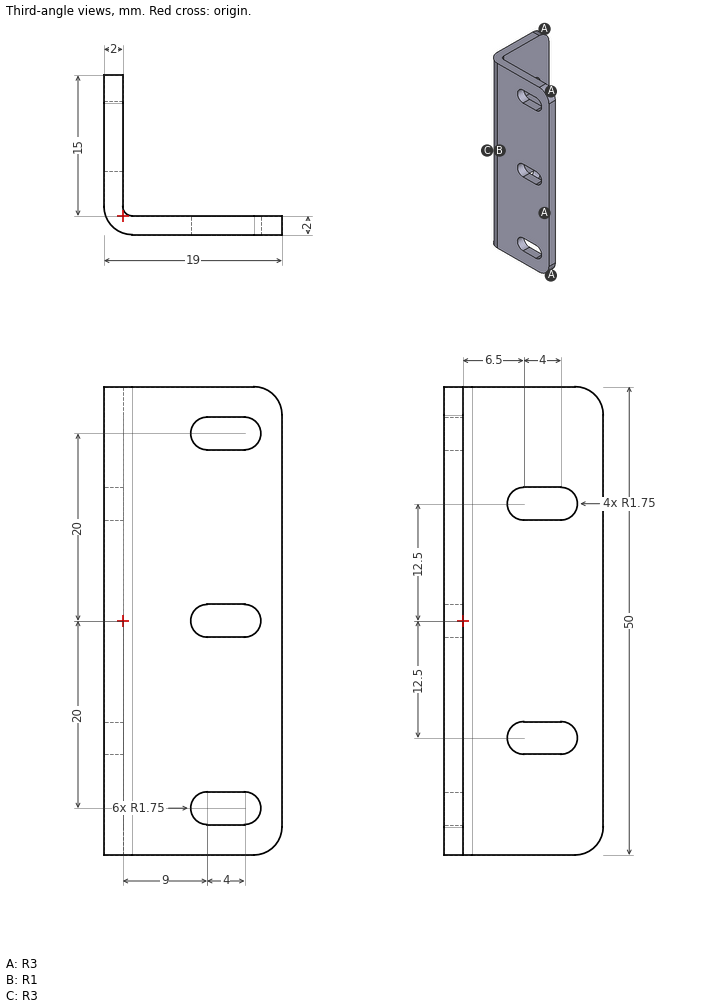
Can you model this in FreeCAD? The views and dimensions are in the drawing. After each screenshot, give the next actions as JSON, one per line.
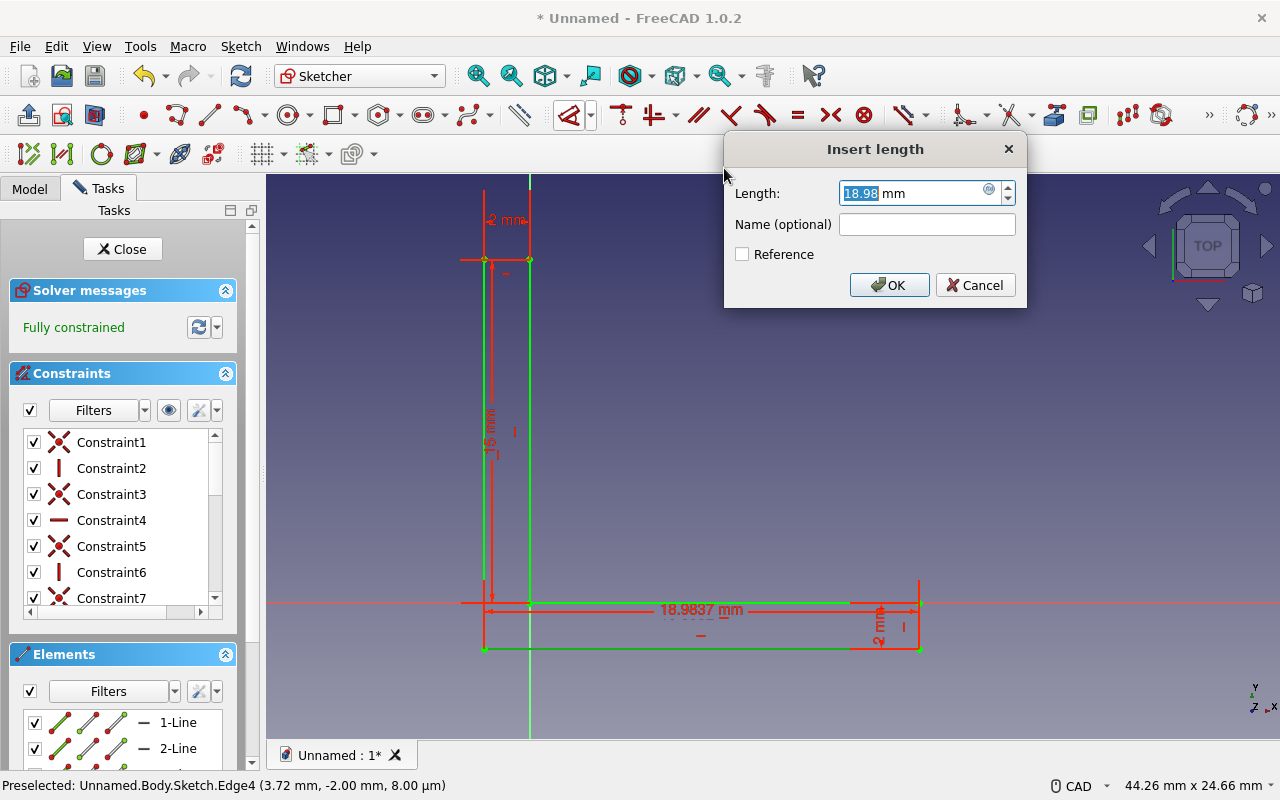
{"action": "type", "text": "19"}
{"action": "key", "text": "Return"}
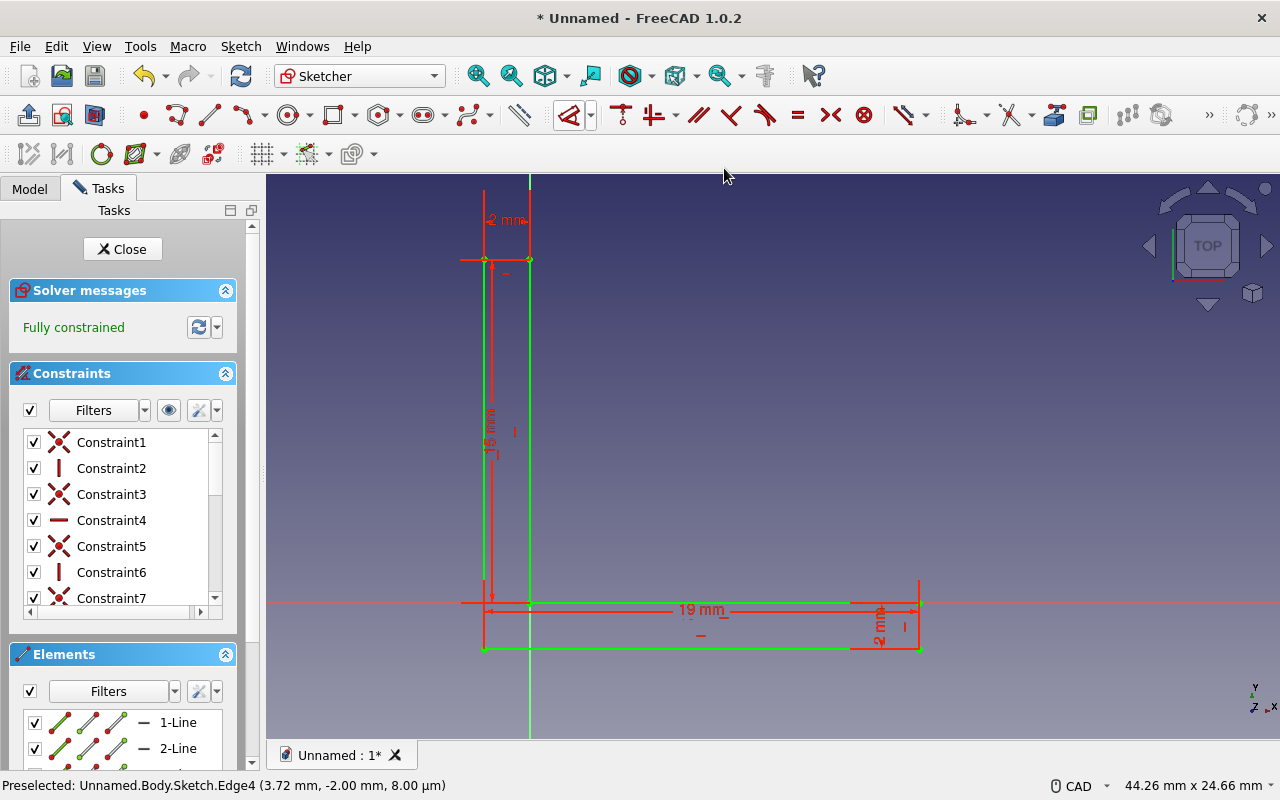
{"action": "left_click", "coordinate": [123, 249]}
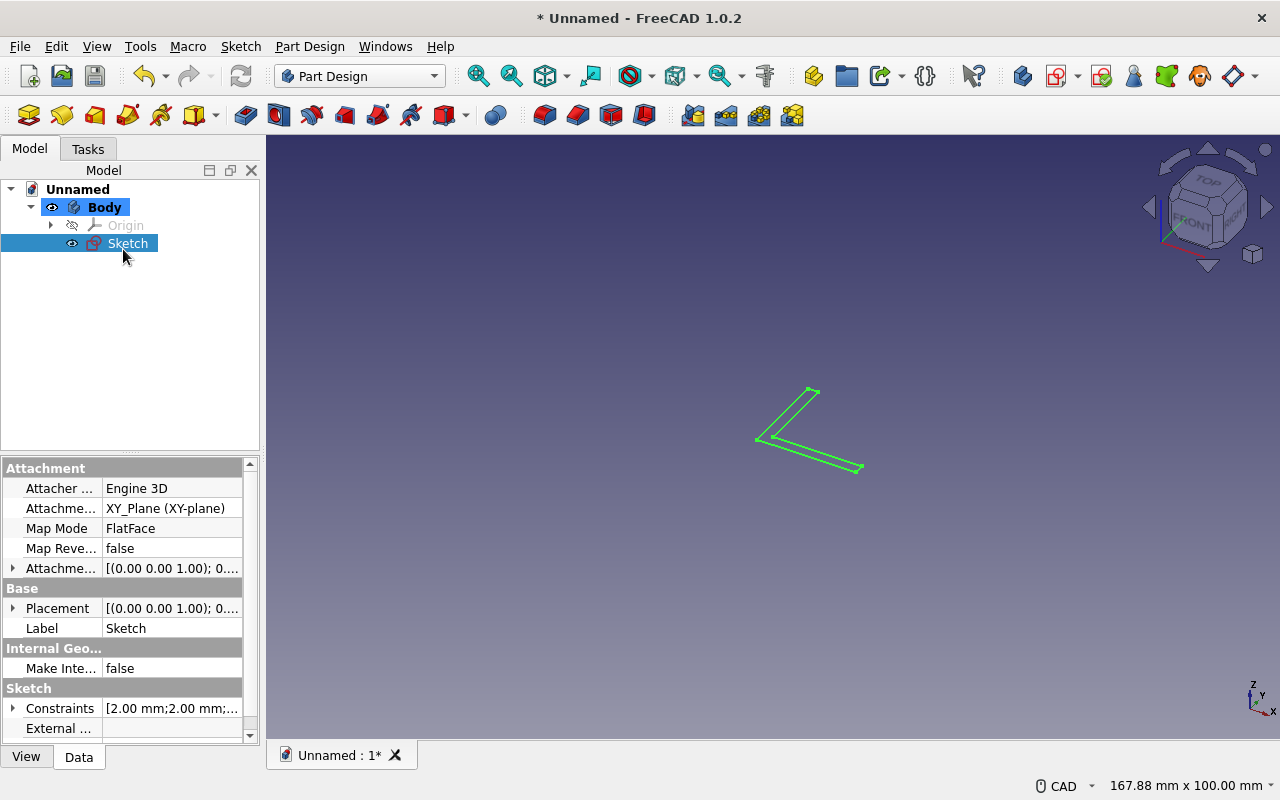
{"action": "left_click", "coordinate": [29, 116]}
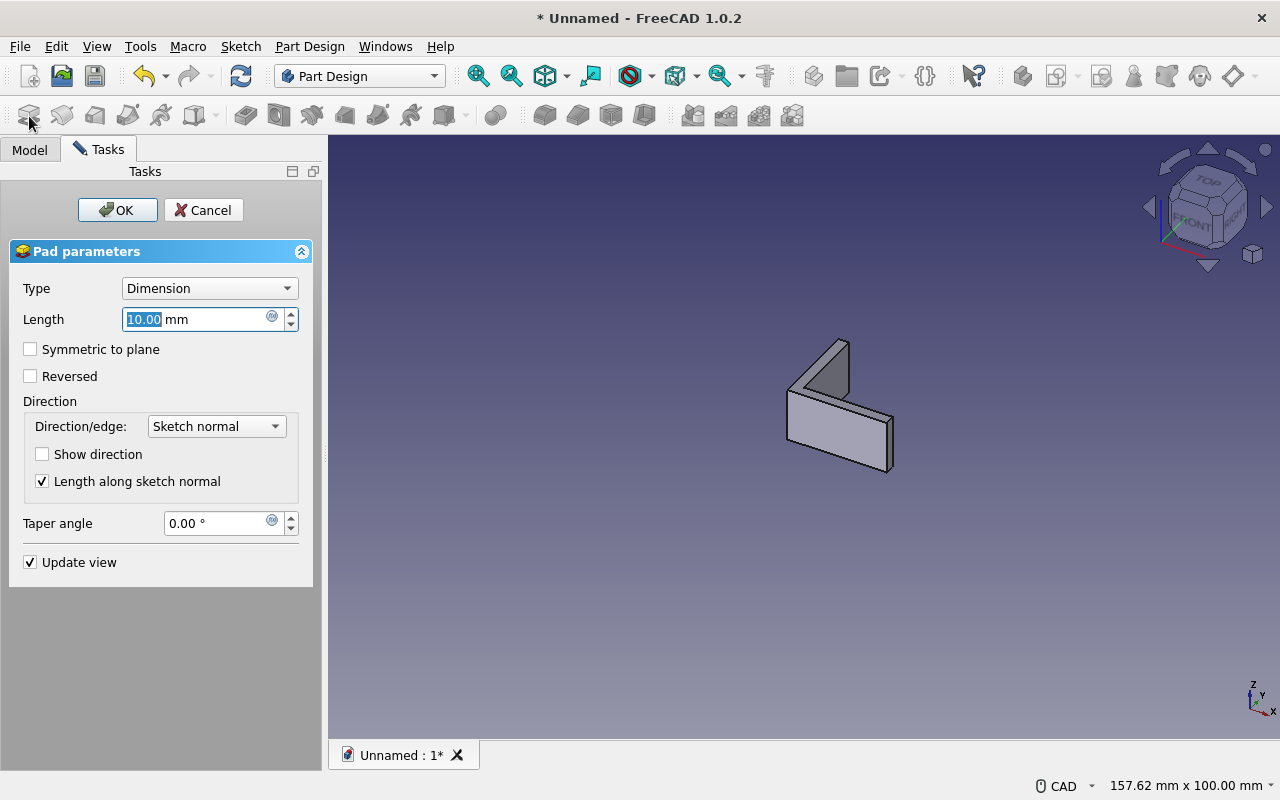
{"action": "type", "text": "50"}
{"action": "key", "text": "Tab"}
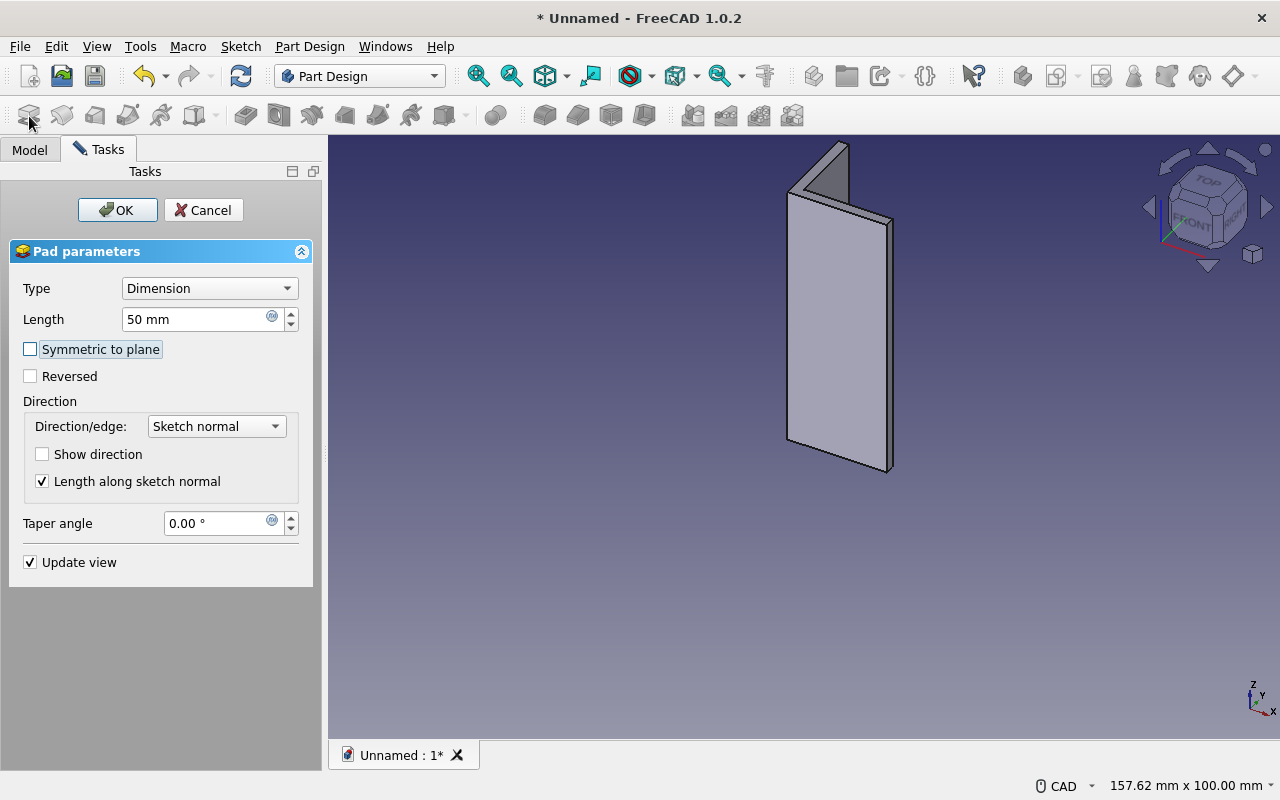
{"action": "left_click", "coordinate": [31, 349]}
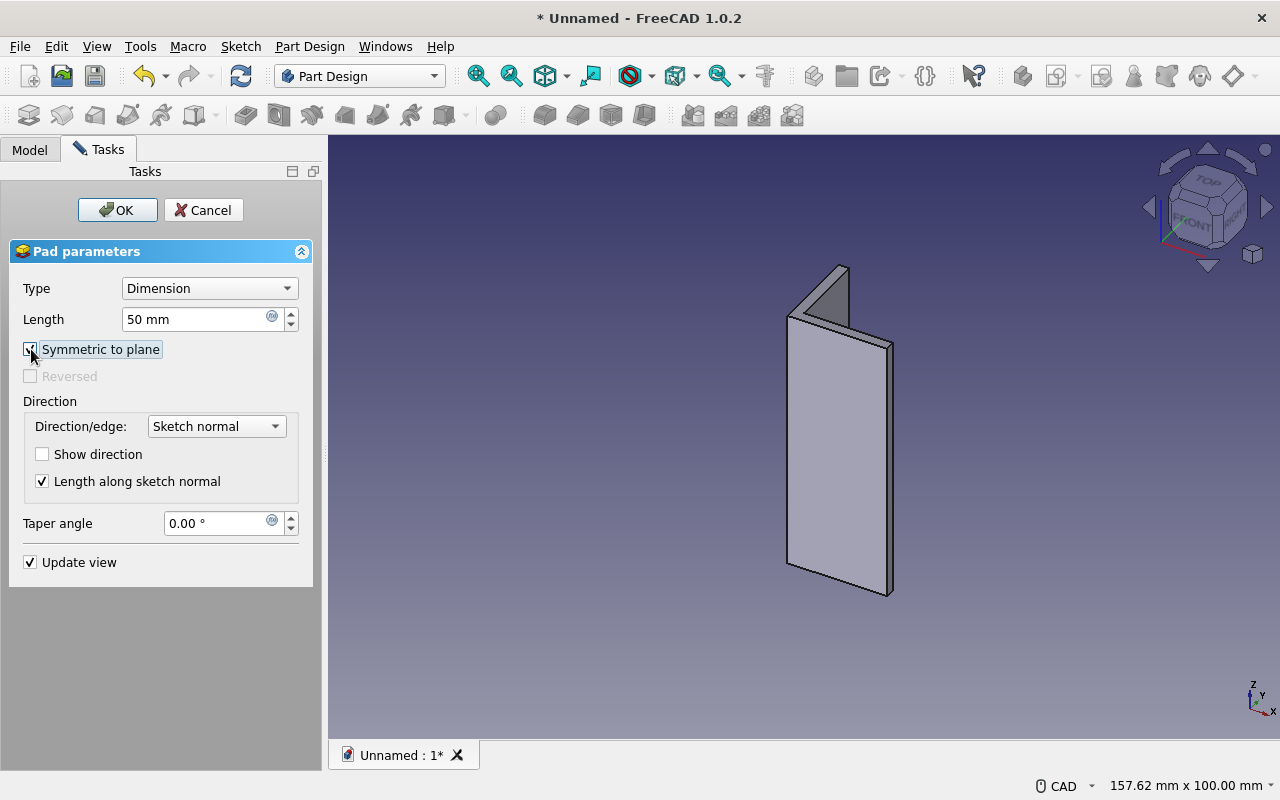
{"action": "left_click", "coordinate": [118, 210]}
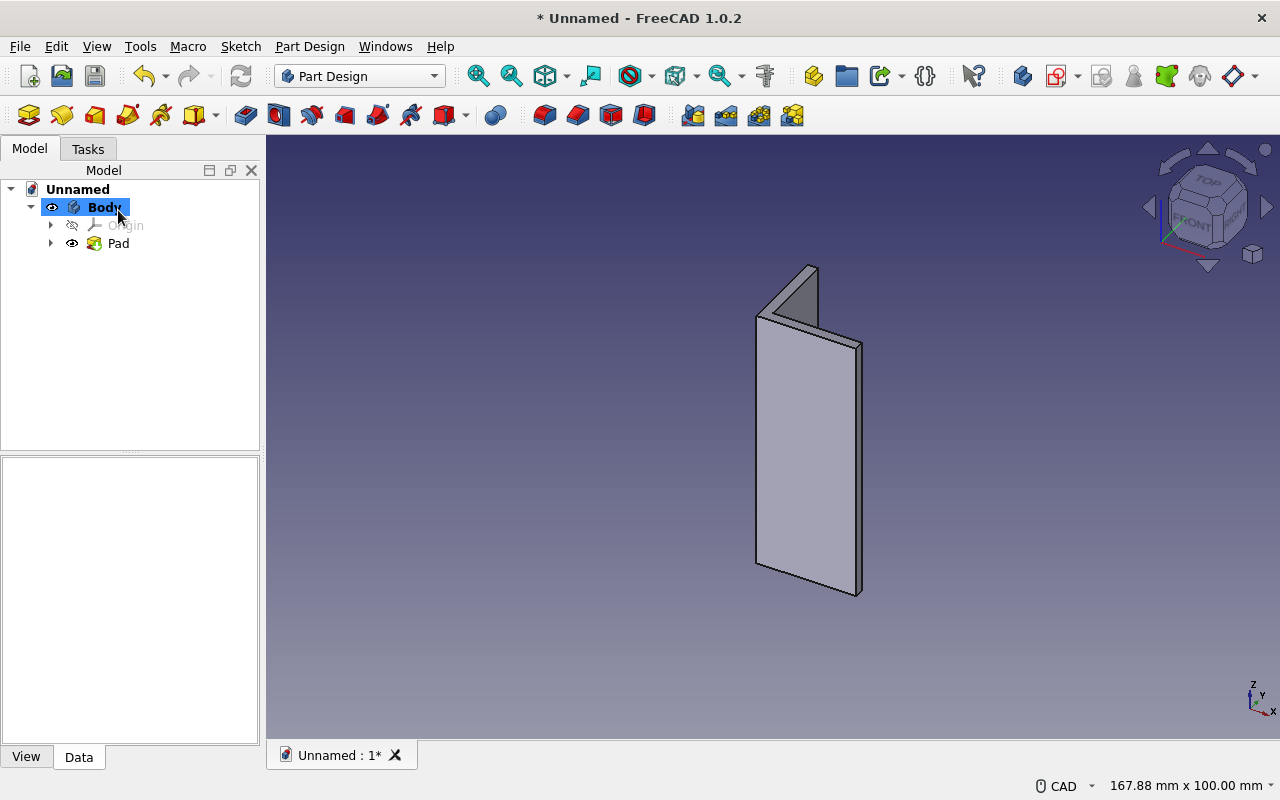
{"action": "key", "text": "4"}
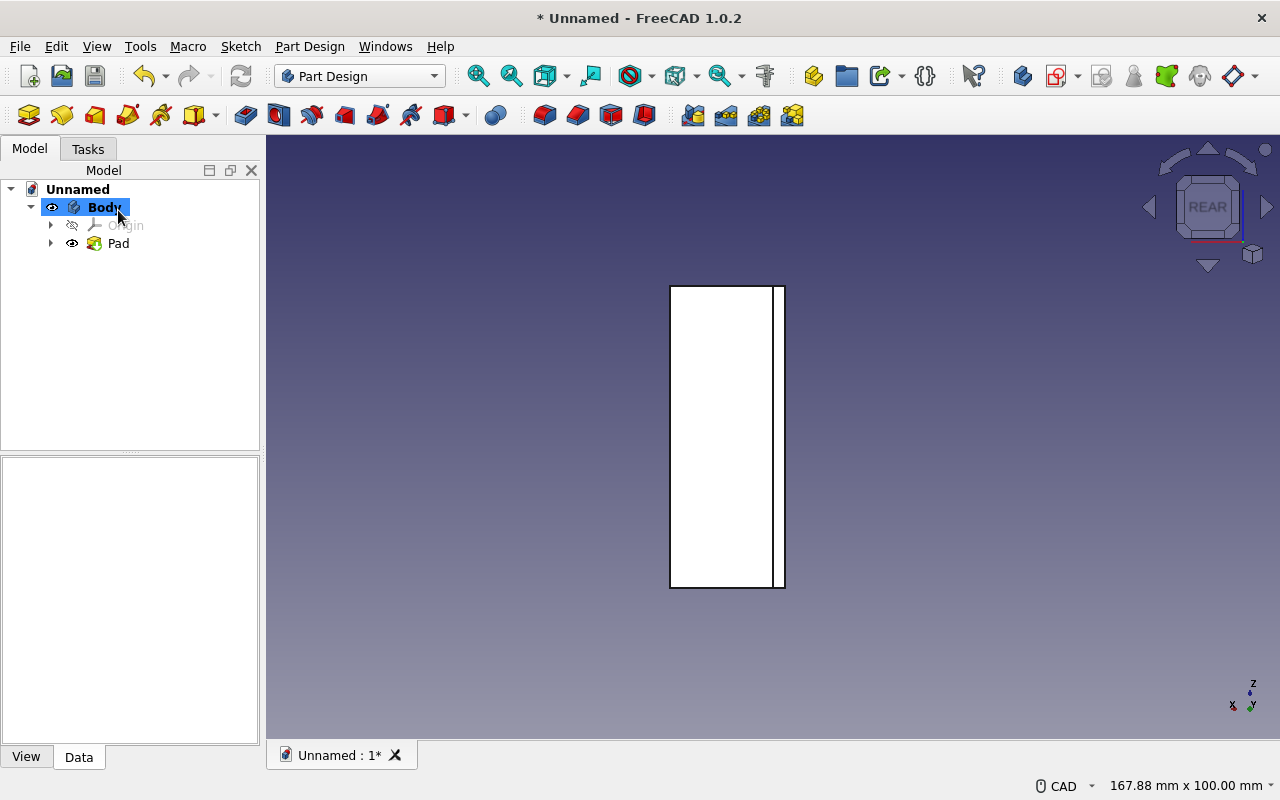
{"action": "left_click", "coordinate": [722, 350]}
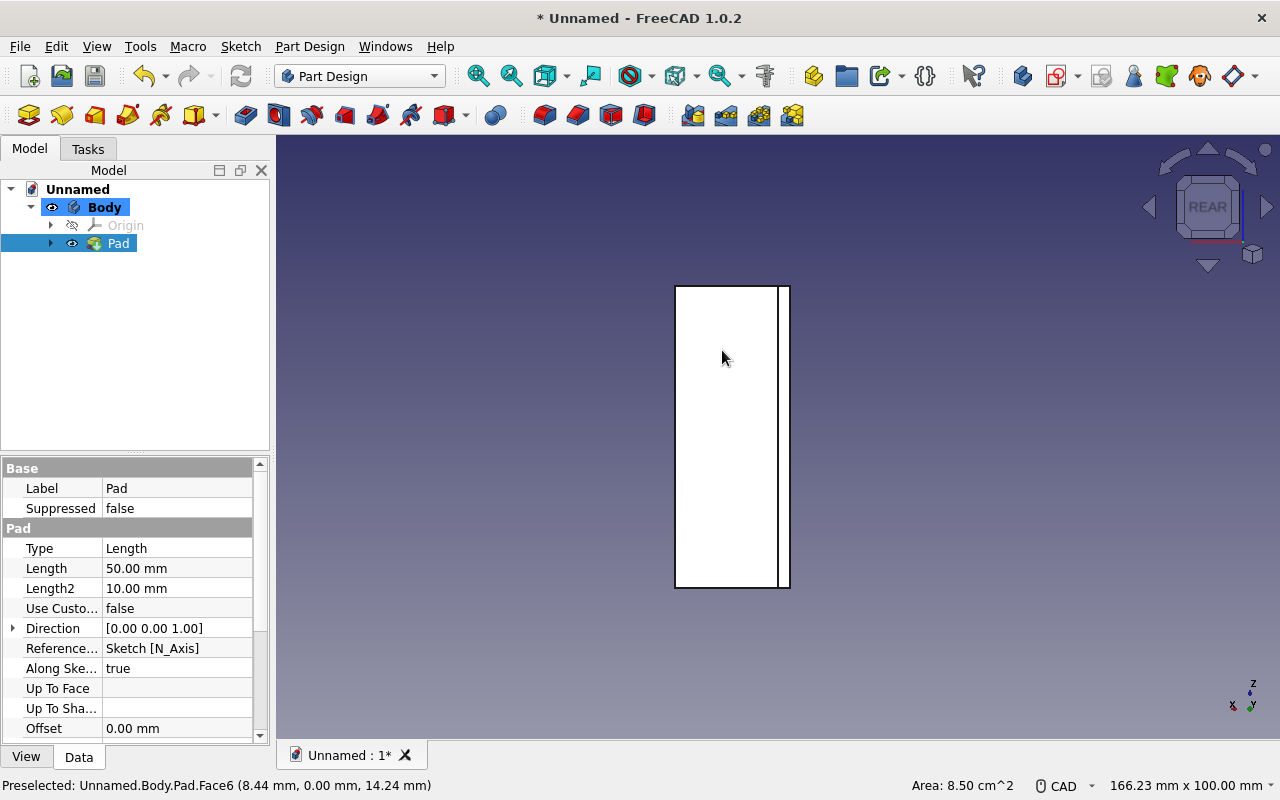
{"action": "left_click", "coordinate": [1056, 76]}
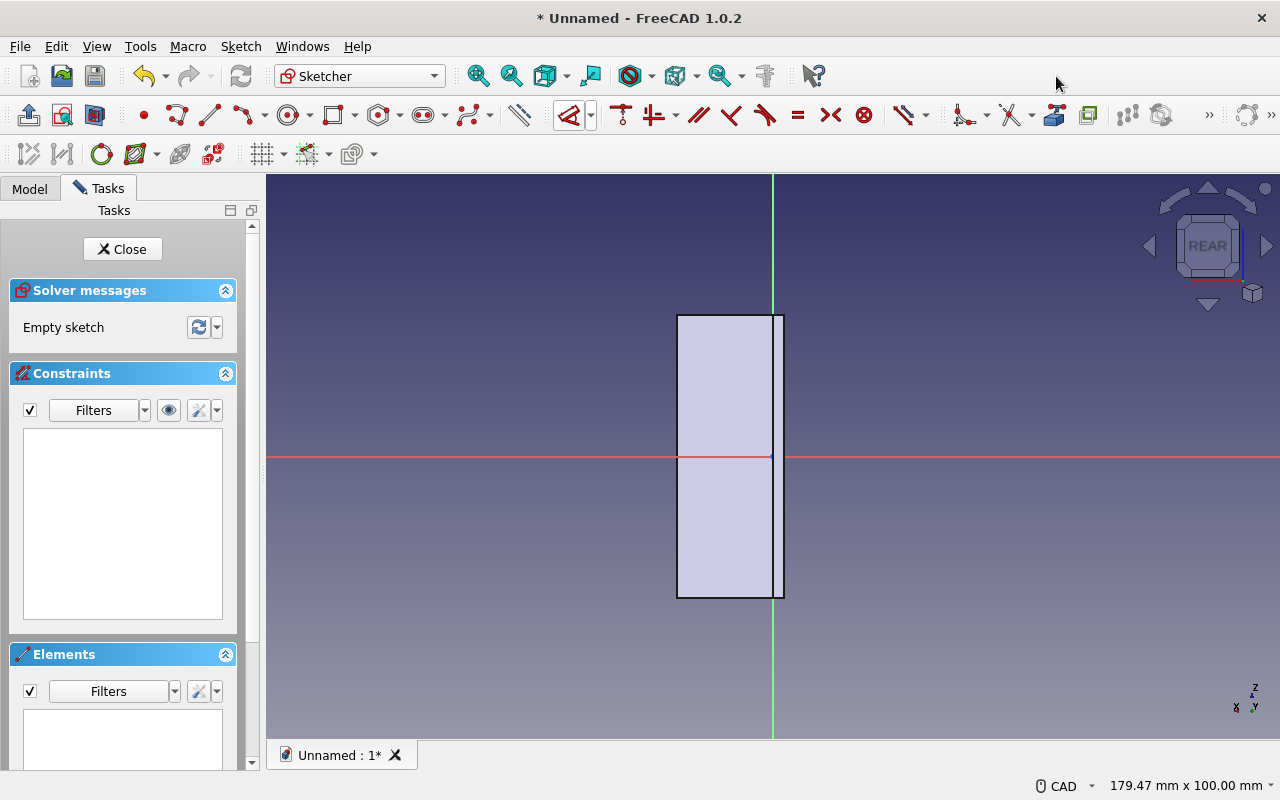
{"action": "left_click", "coordinate": [95, 116]}